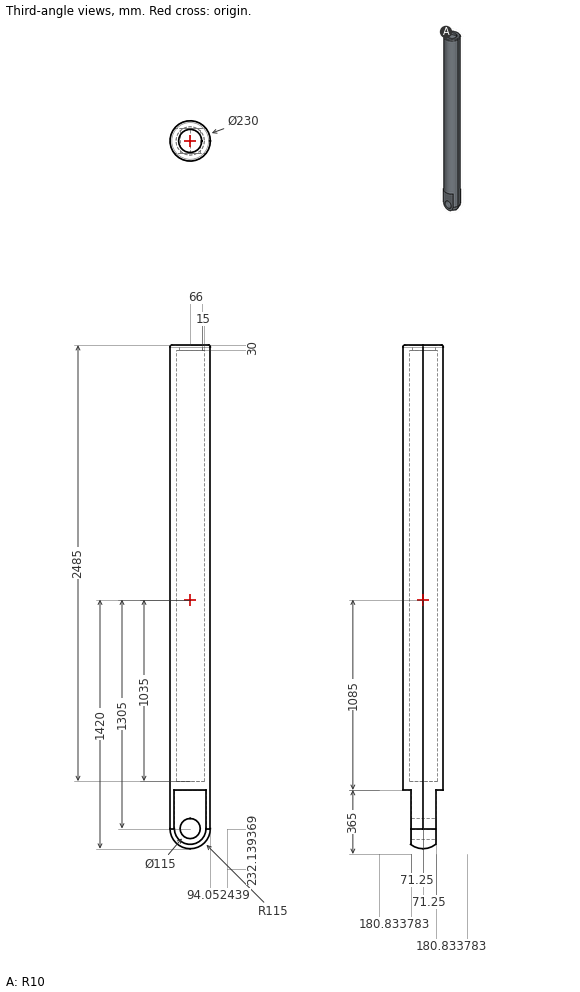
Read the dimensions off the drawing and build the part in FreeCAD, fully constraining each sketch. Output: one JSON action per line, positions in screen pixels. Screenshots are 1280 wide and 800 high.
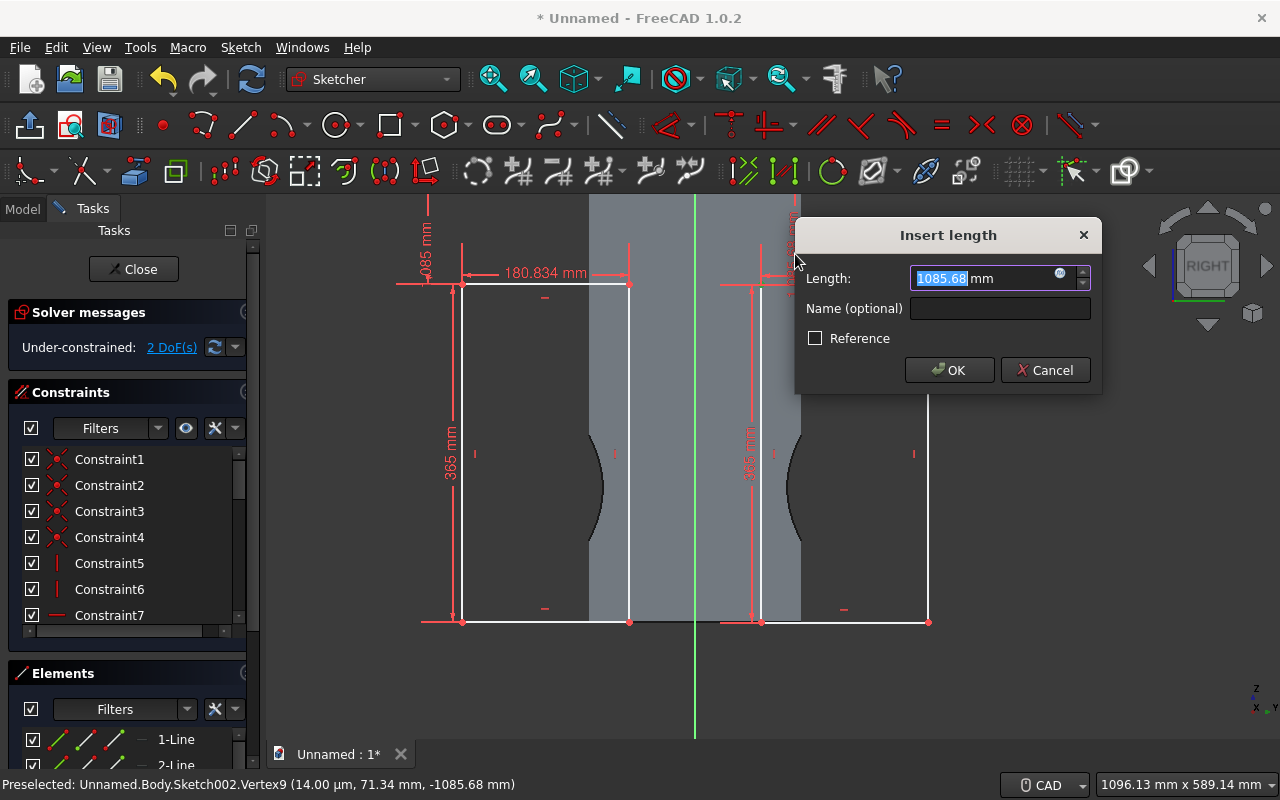
{"action": "type", "text": "1085"}
{"action": "key", "text": "Return"}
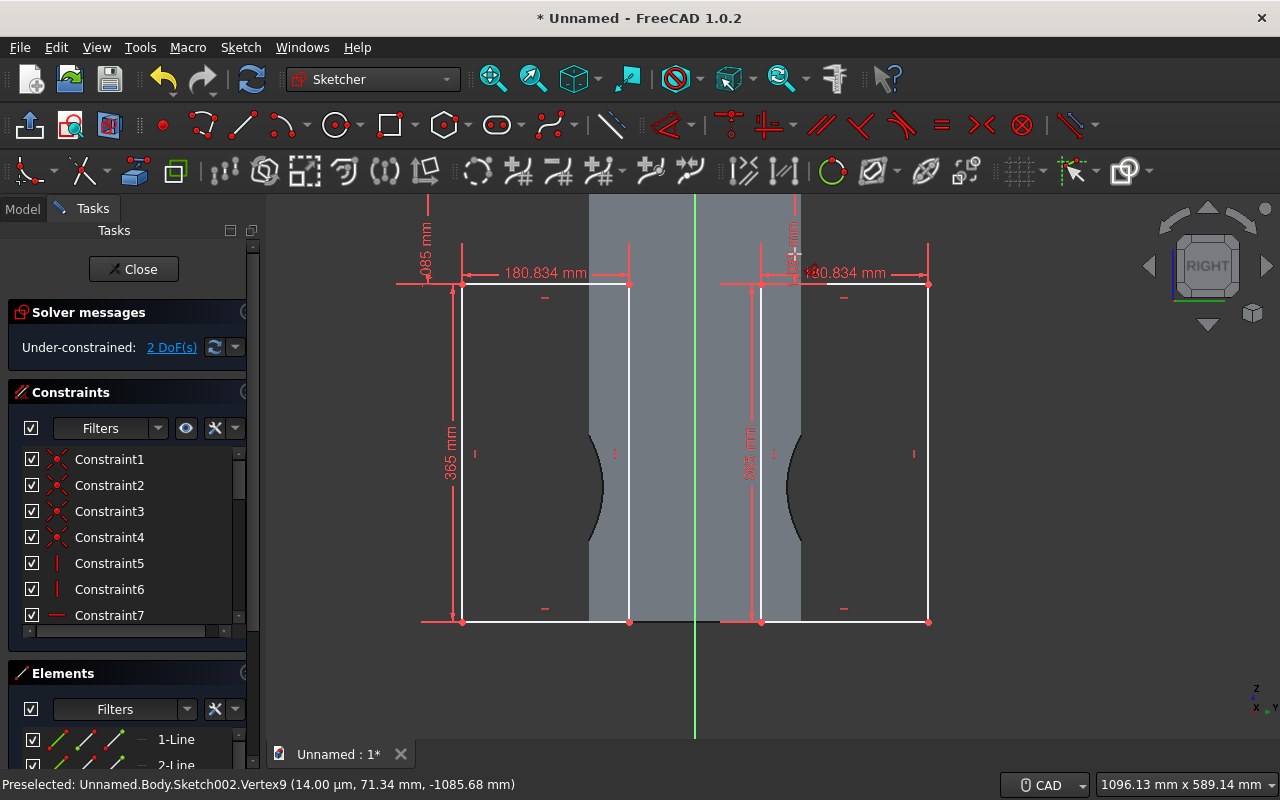
{"action": "left_click", "coordinate": [629, 622]}
{"action": "left_click", "coordinate": [662, 656]}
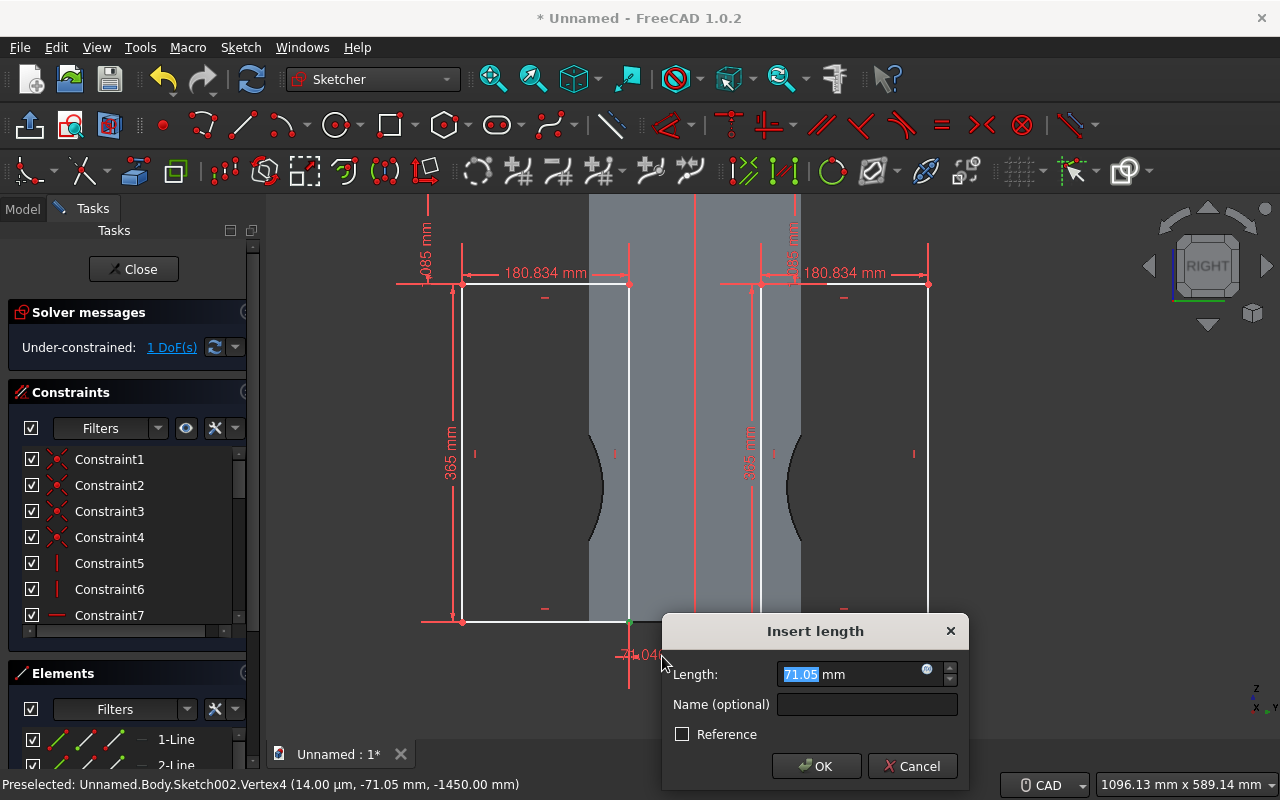
{"action": "type", "text": "71.25"}
{"action": "key", "text": "Return"}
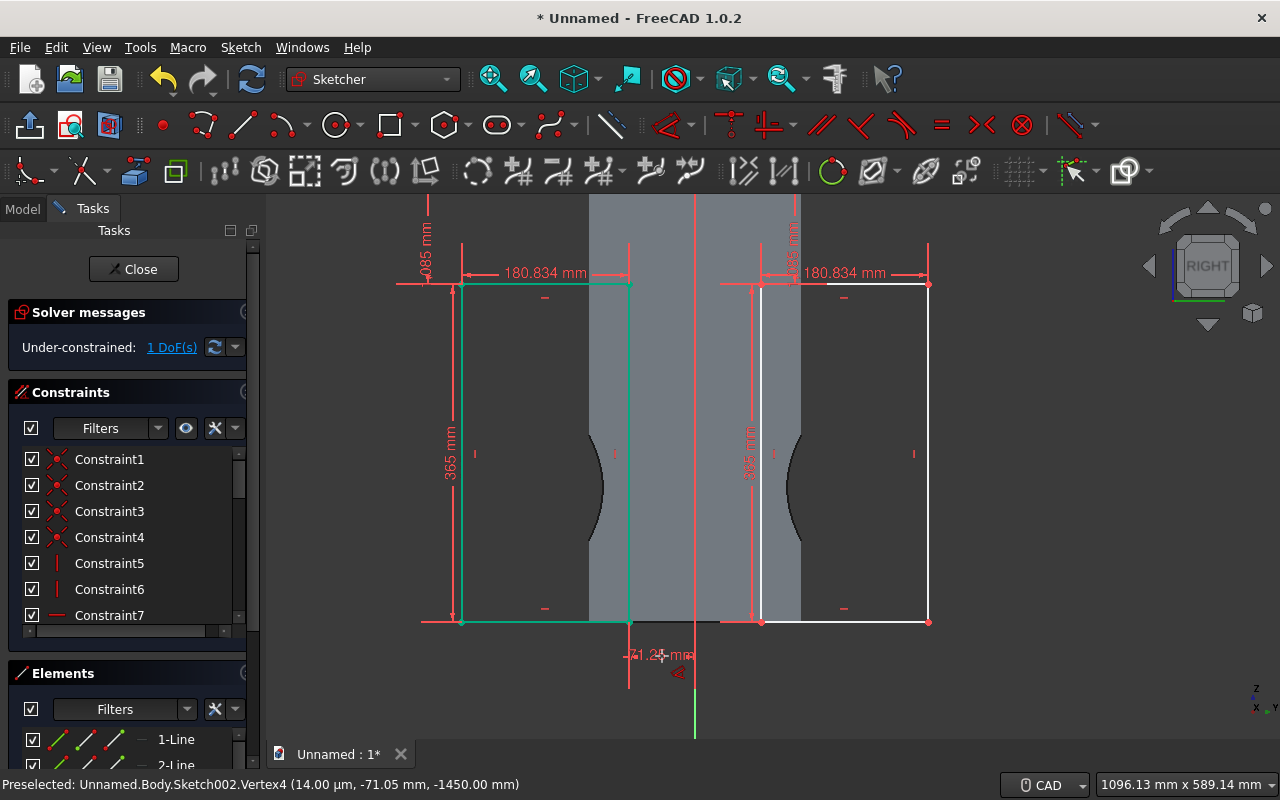
{"action": "left_click", "coordinate": [761, 284]}
{"action": "left_click", "coordinate": [728, 318]}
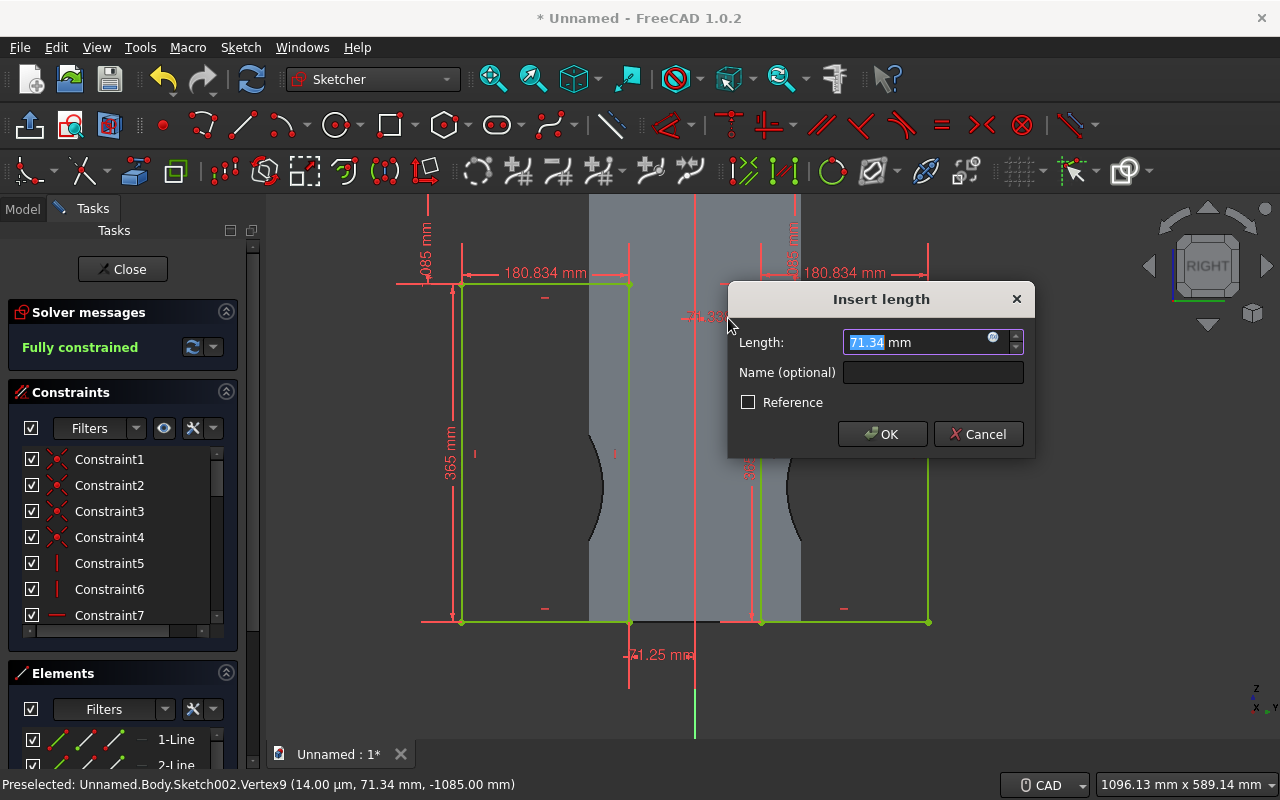
{"action": "type", "text": "71.25"}
{"action": "key", "text": "Return"}
{"action": "key", "text": "Escape"}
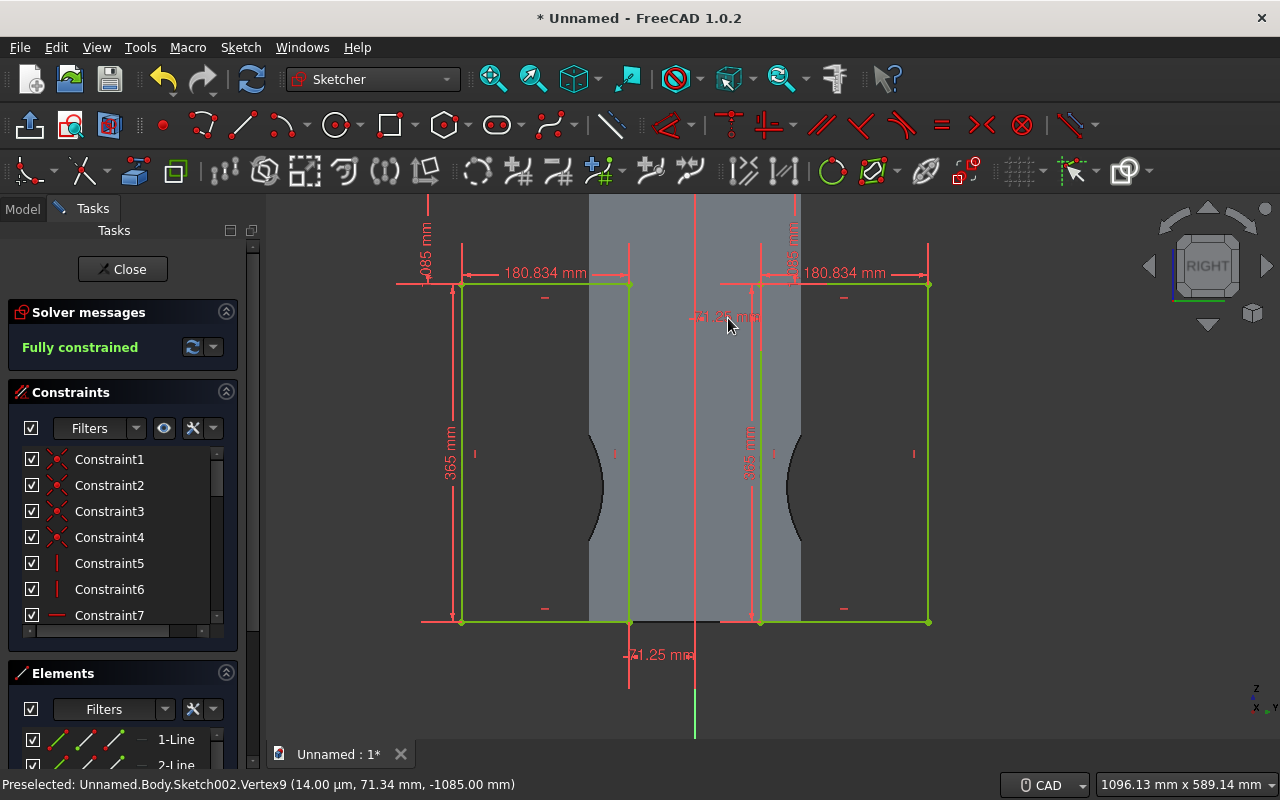
{"action": "left_click", "coordinate": [123, 269]}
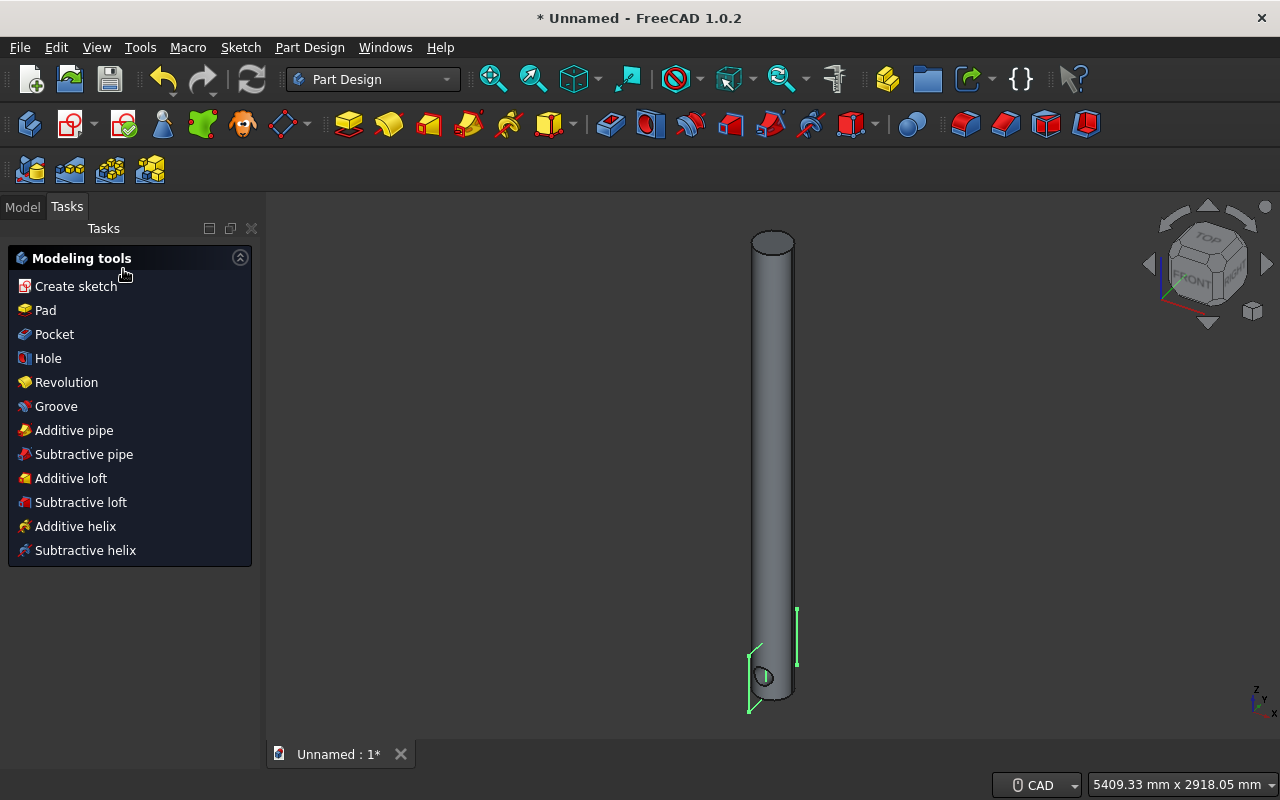
{"action": "left_click", "coordinate": [612, 124]}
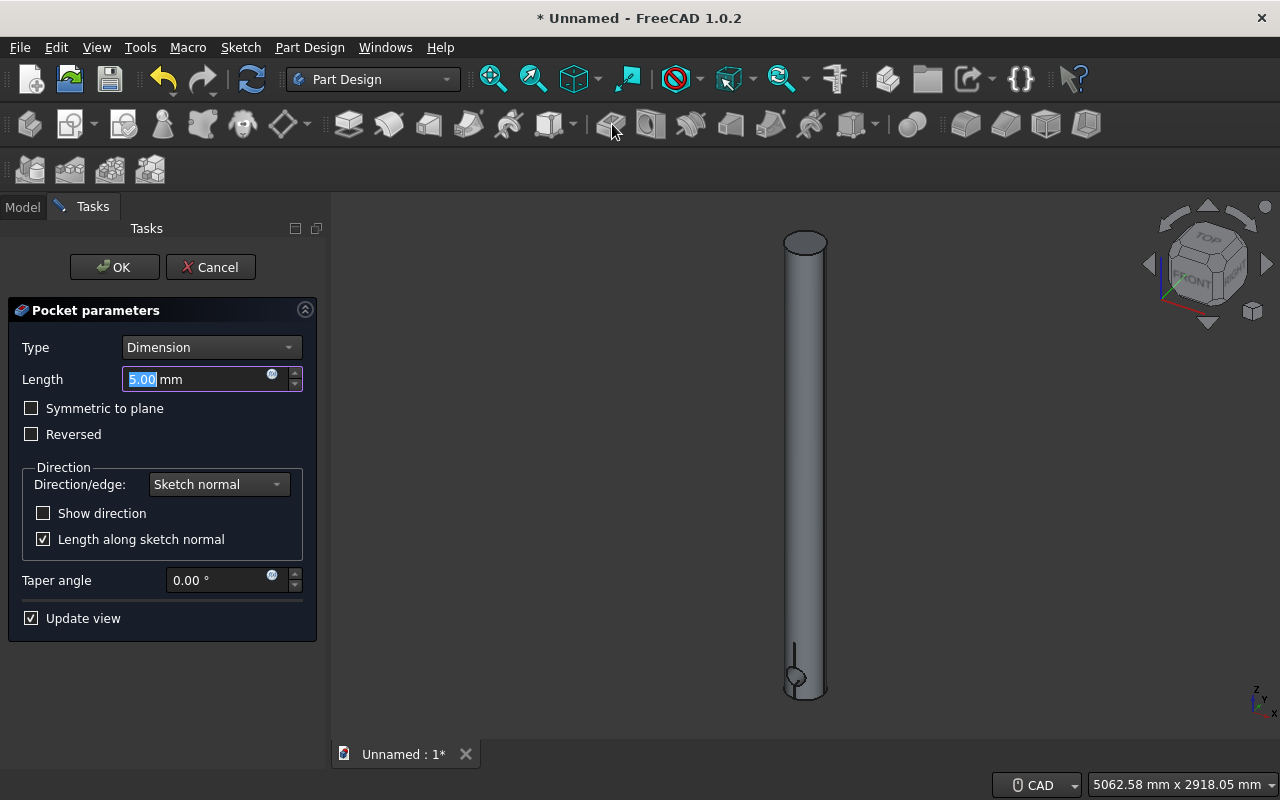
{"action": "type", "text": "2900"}
{"action": "key", "text": "Tab"}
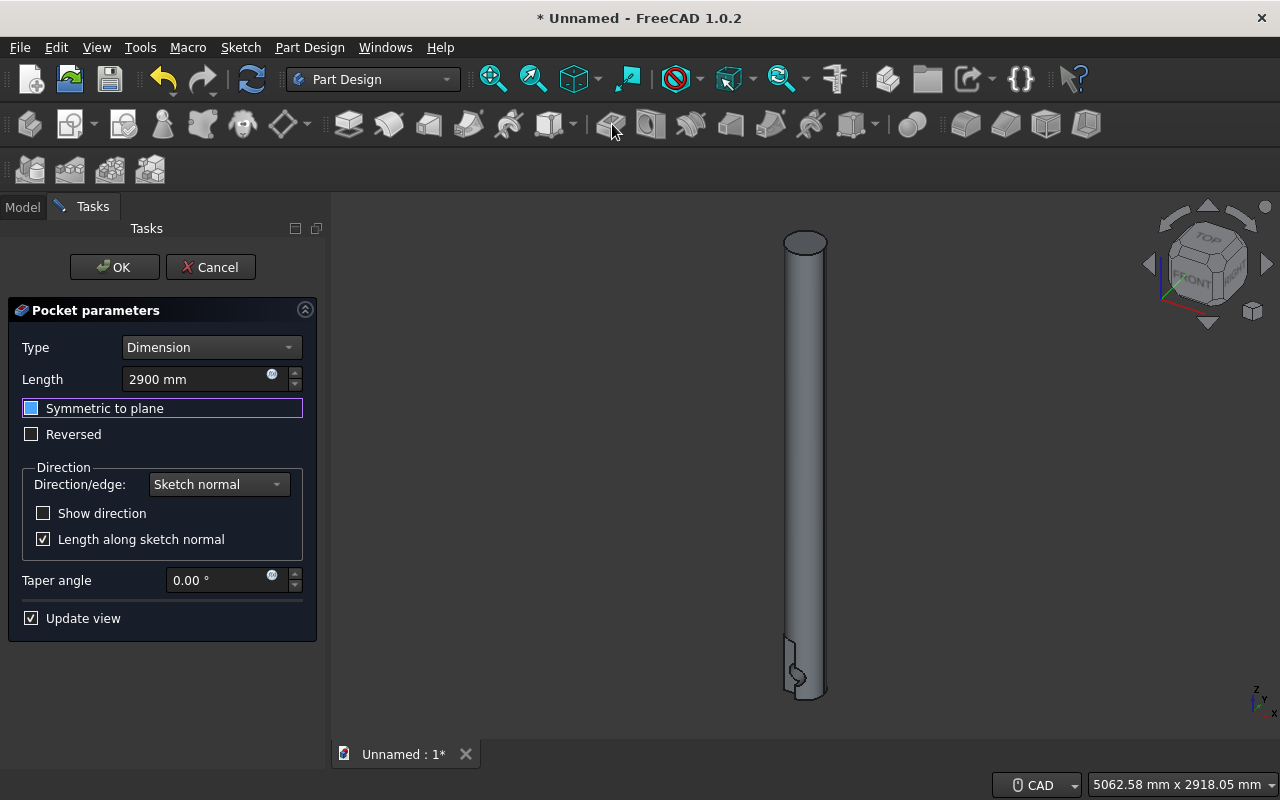
{"action": "left_click", "coordinate": [30, 408]}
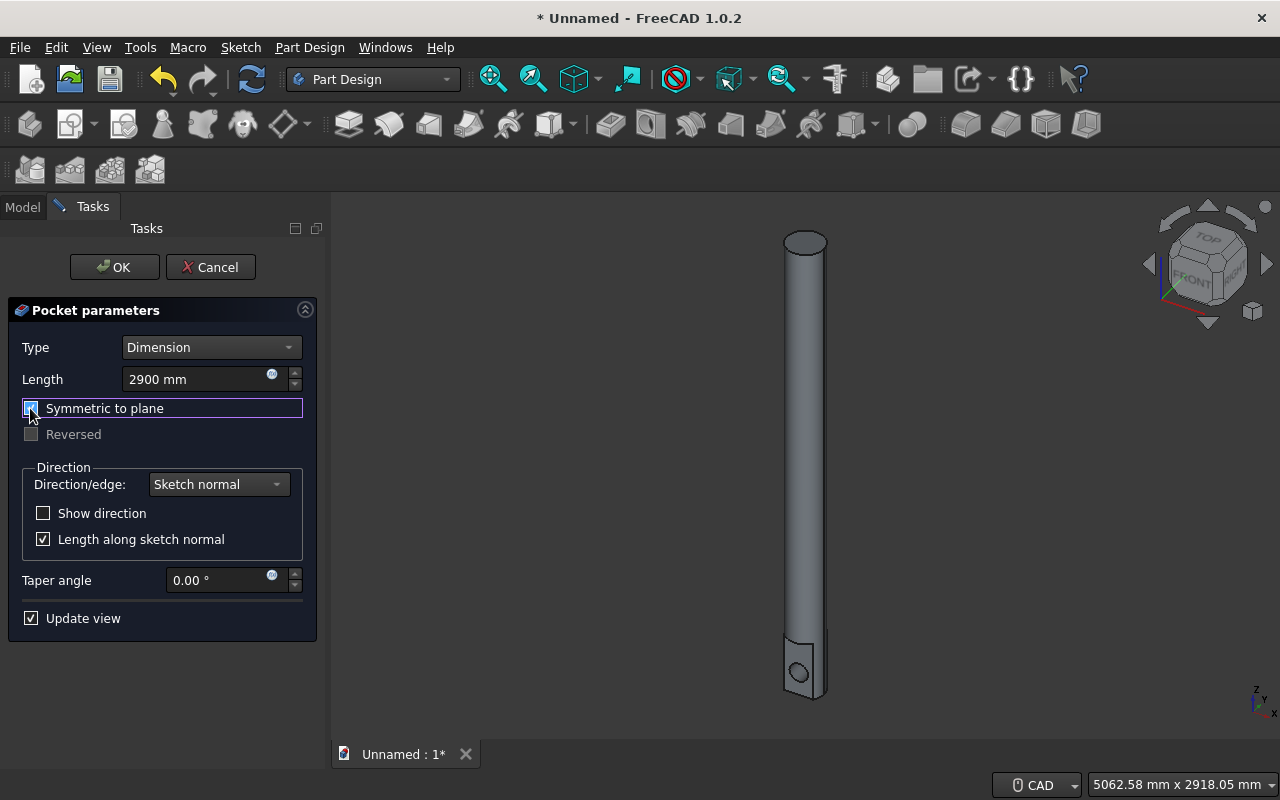
{"action": "left_click", "coordinate": [115, 267]}